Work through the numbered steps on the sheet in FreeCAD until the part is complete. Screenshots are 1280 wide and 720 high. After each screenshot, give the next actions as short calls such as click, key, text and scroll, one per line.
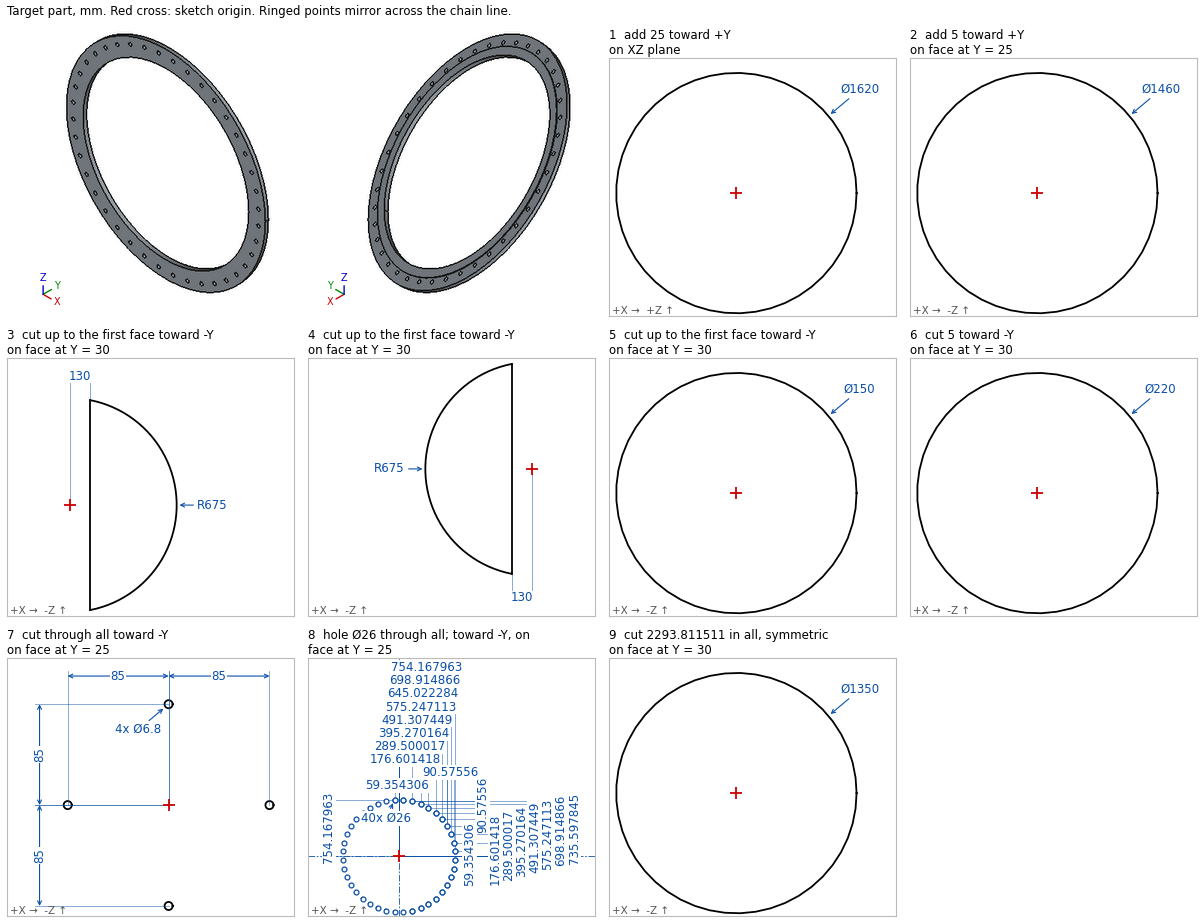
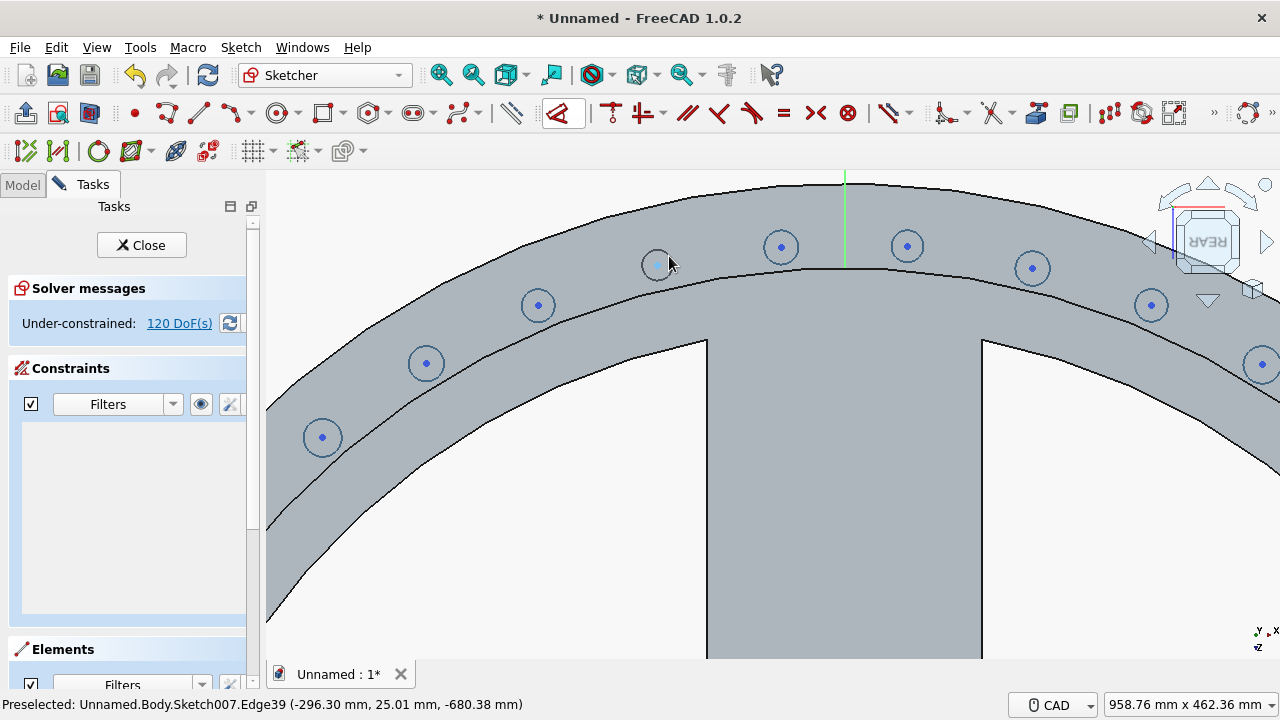
click(668, 254)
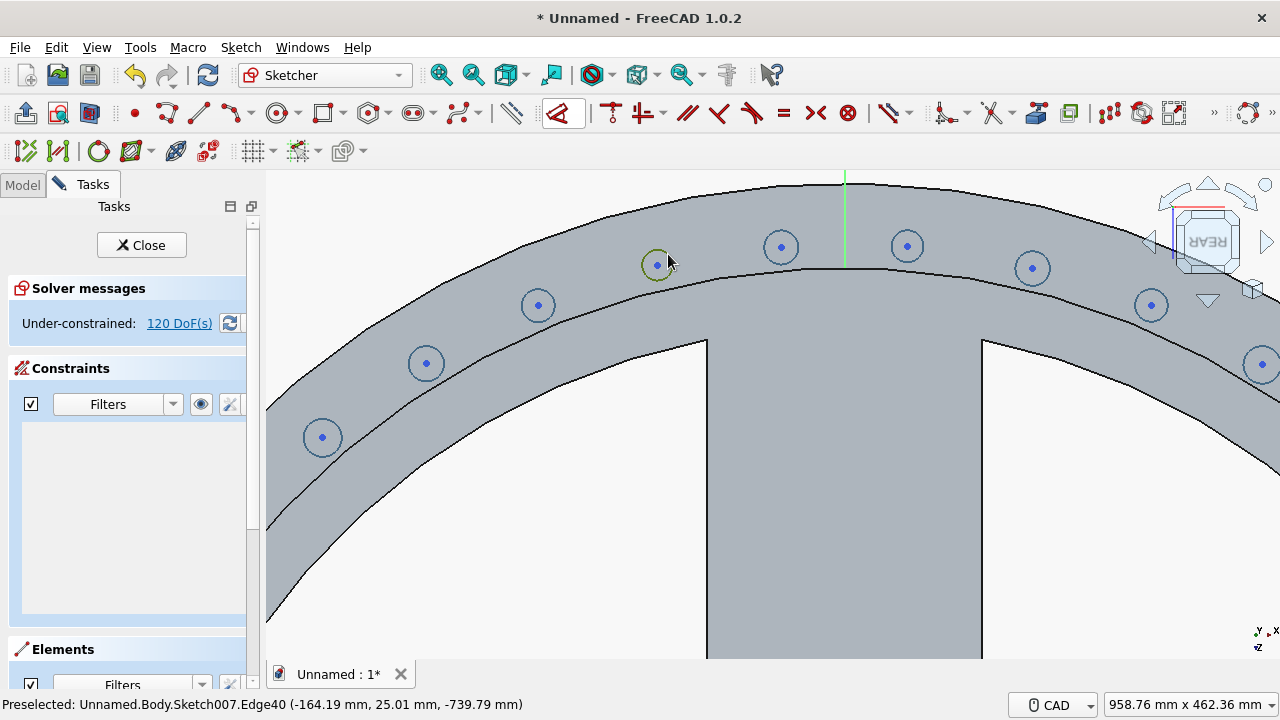
click(784, 114)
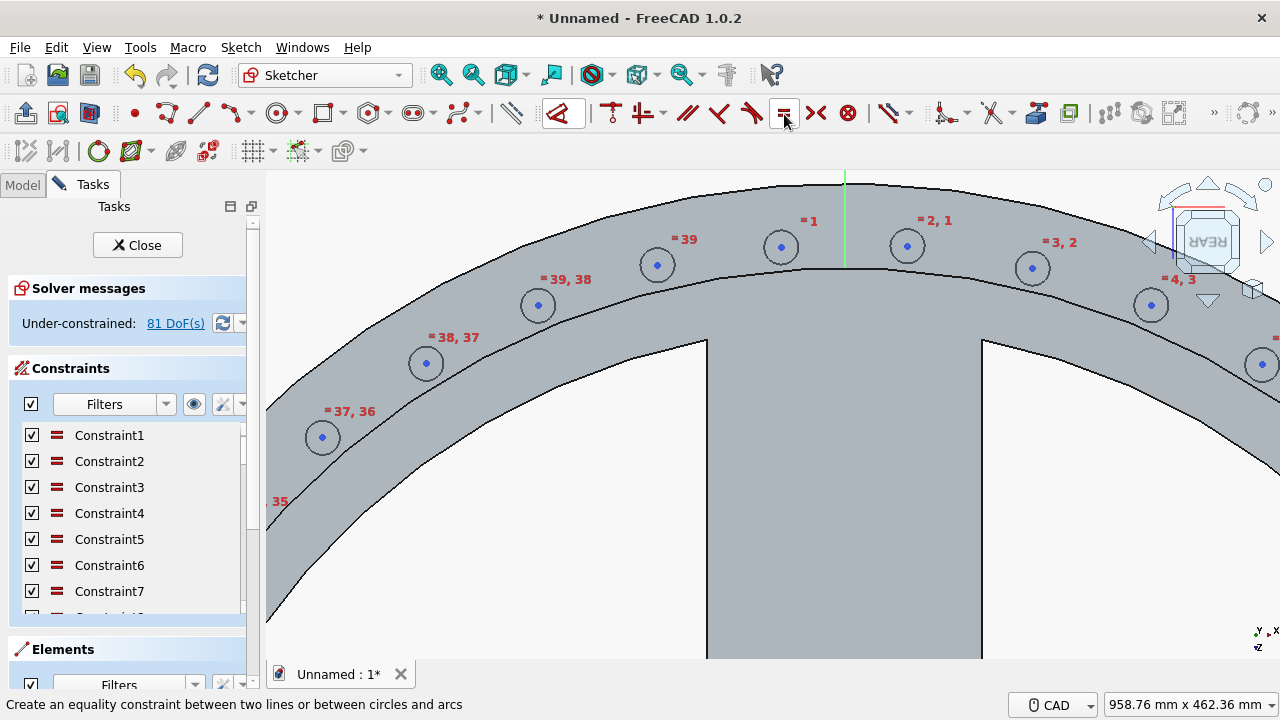
scroll(669, 256, down, 8)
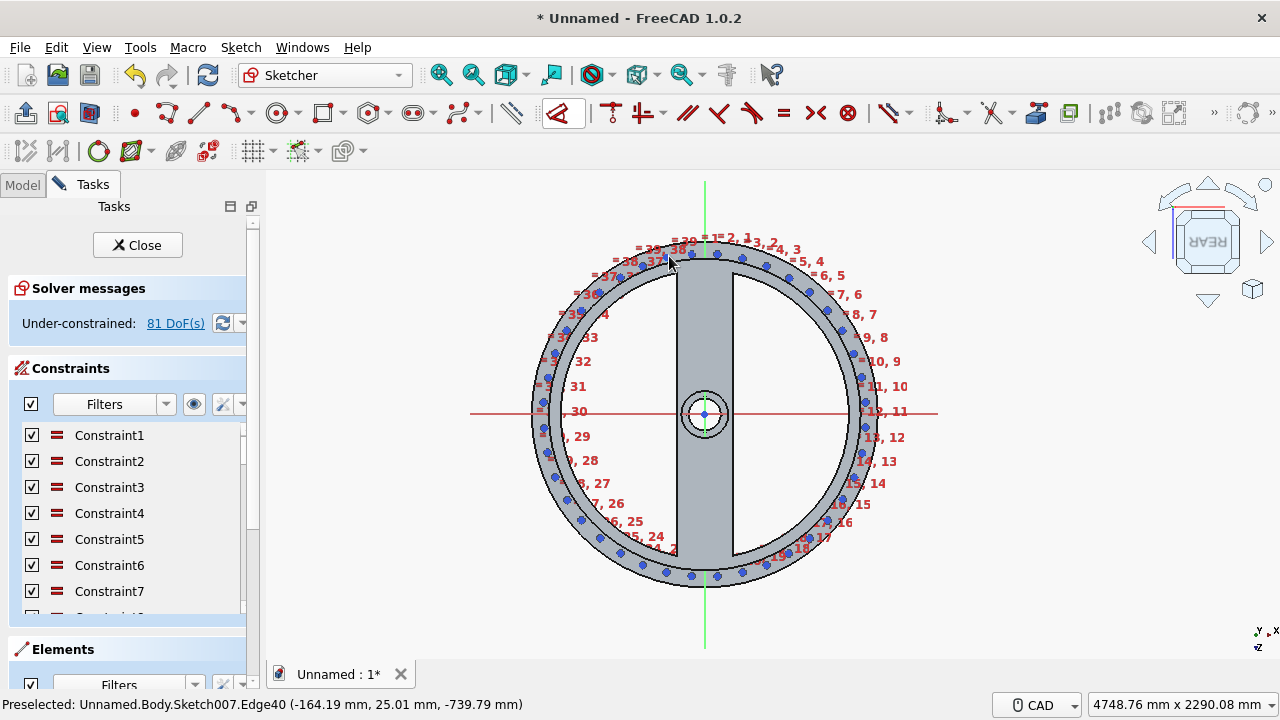
click(692, 254)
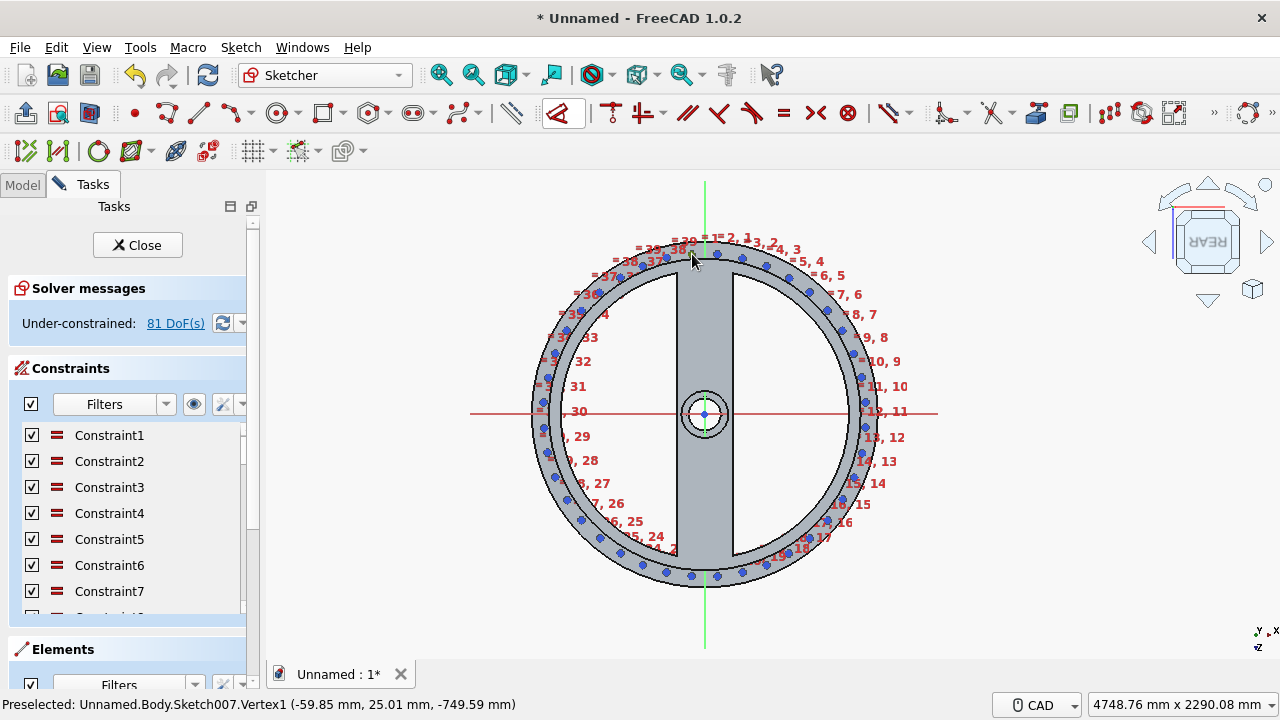
click(717, 254)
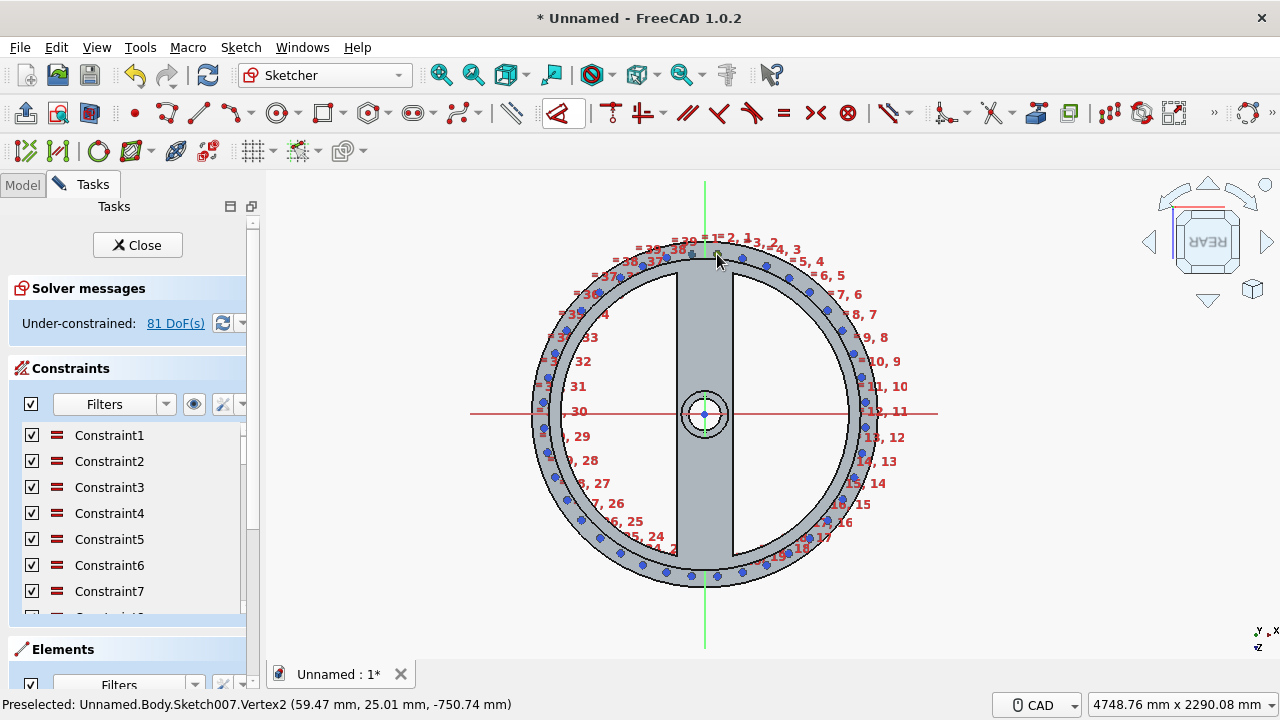
click(705, 538)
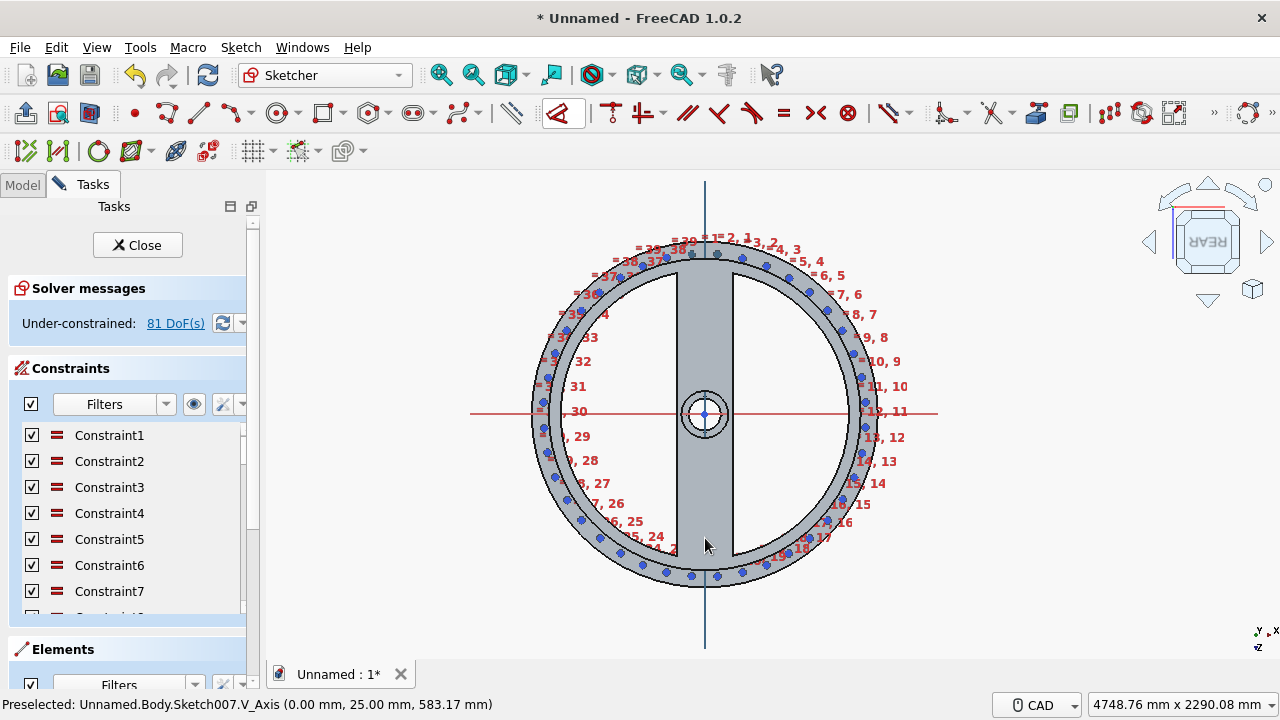
key(s)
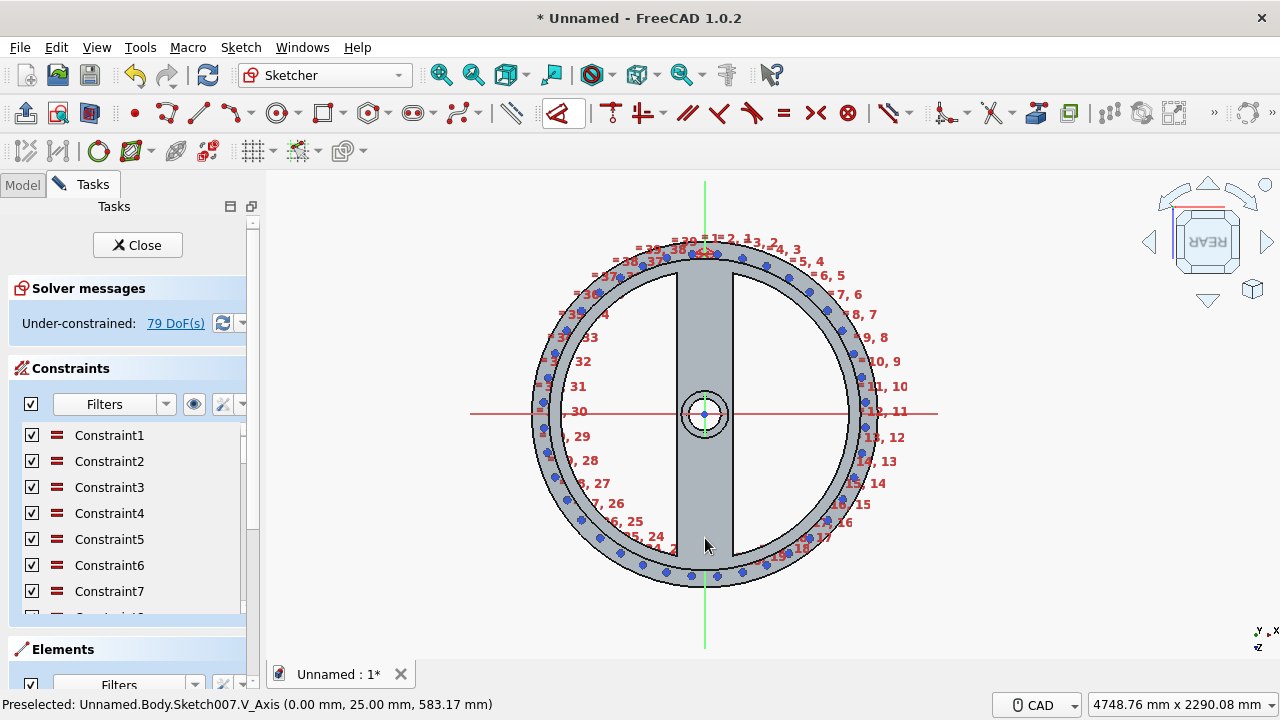
click(866, 402)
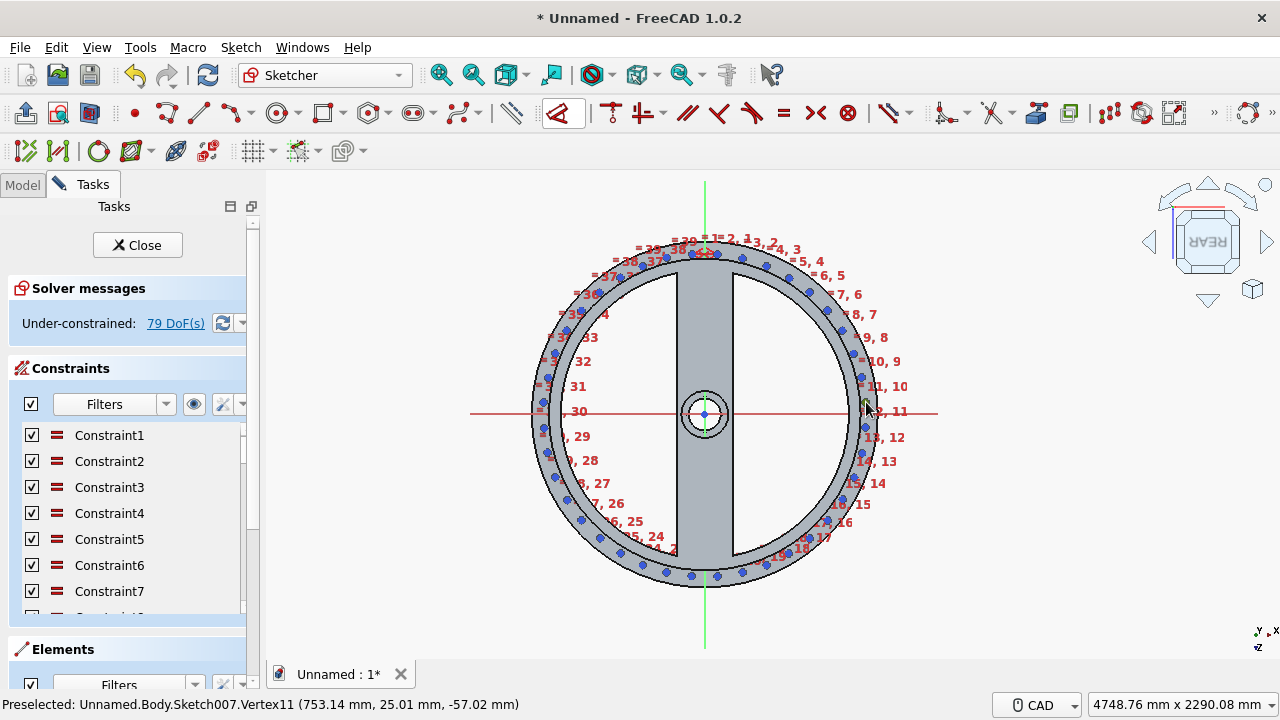
click(866, 428)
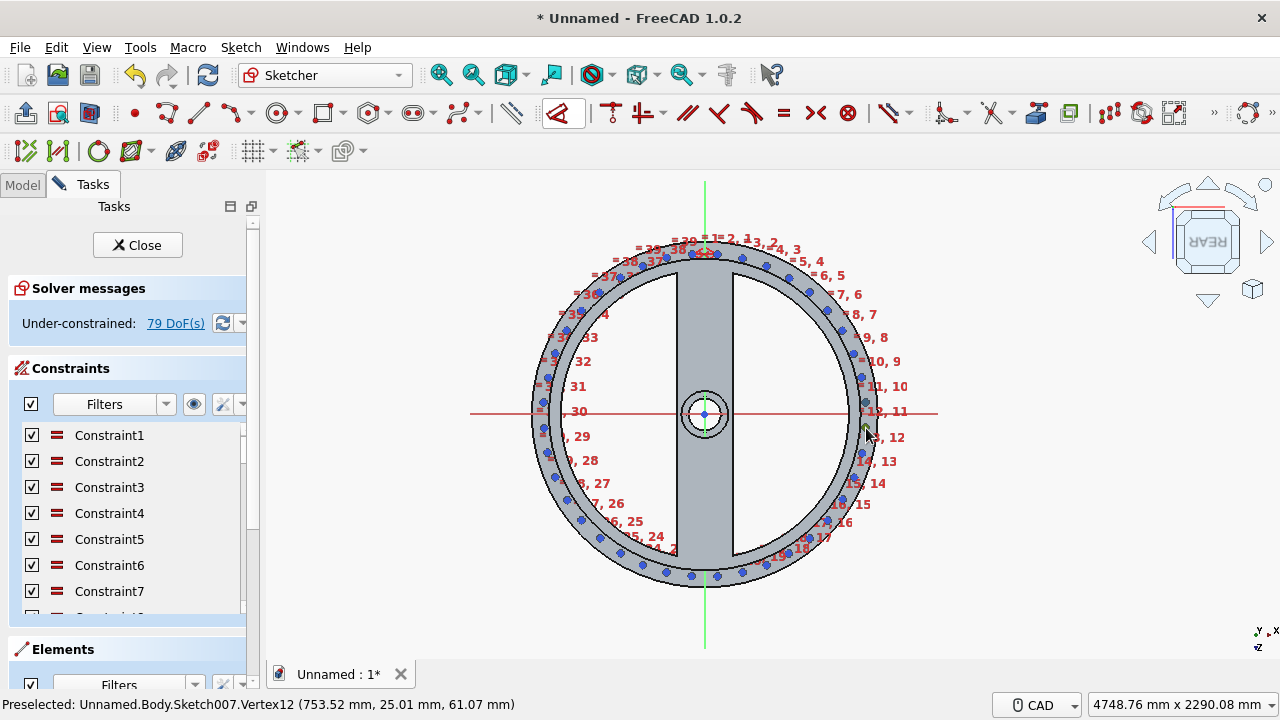
click(470, 414)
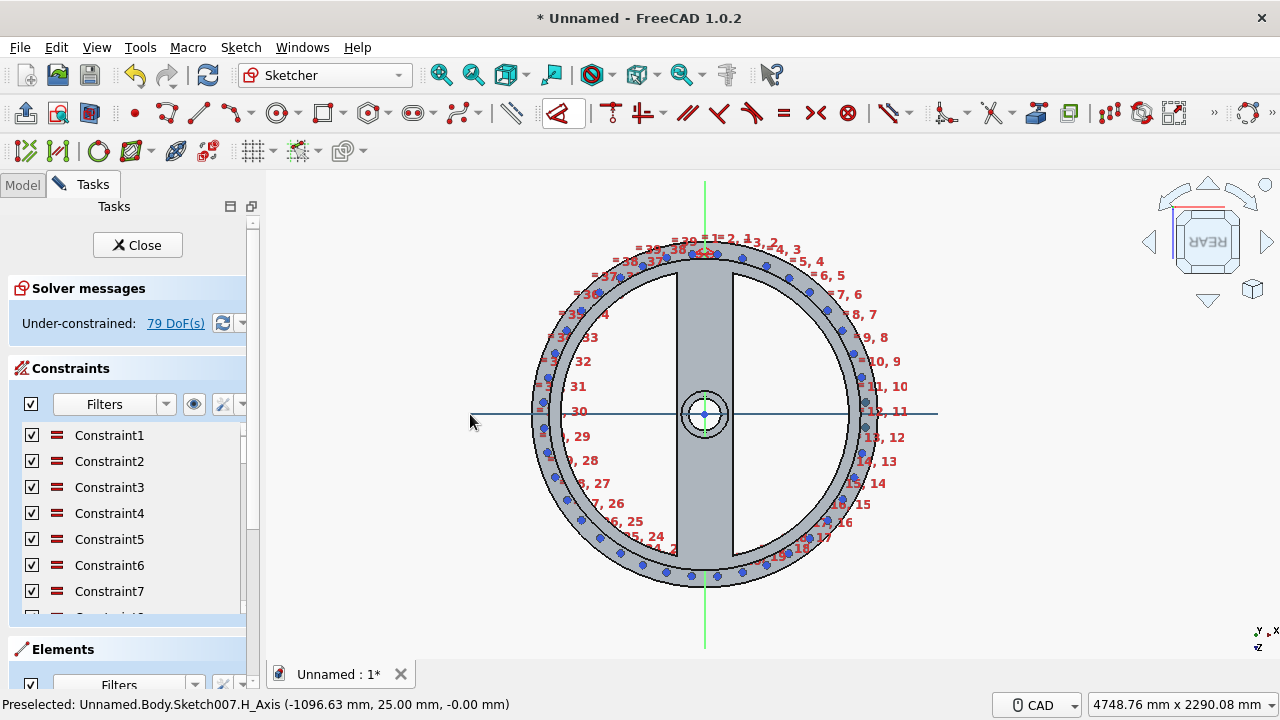
click(816, 114)